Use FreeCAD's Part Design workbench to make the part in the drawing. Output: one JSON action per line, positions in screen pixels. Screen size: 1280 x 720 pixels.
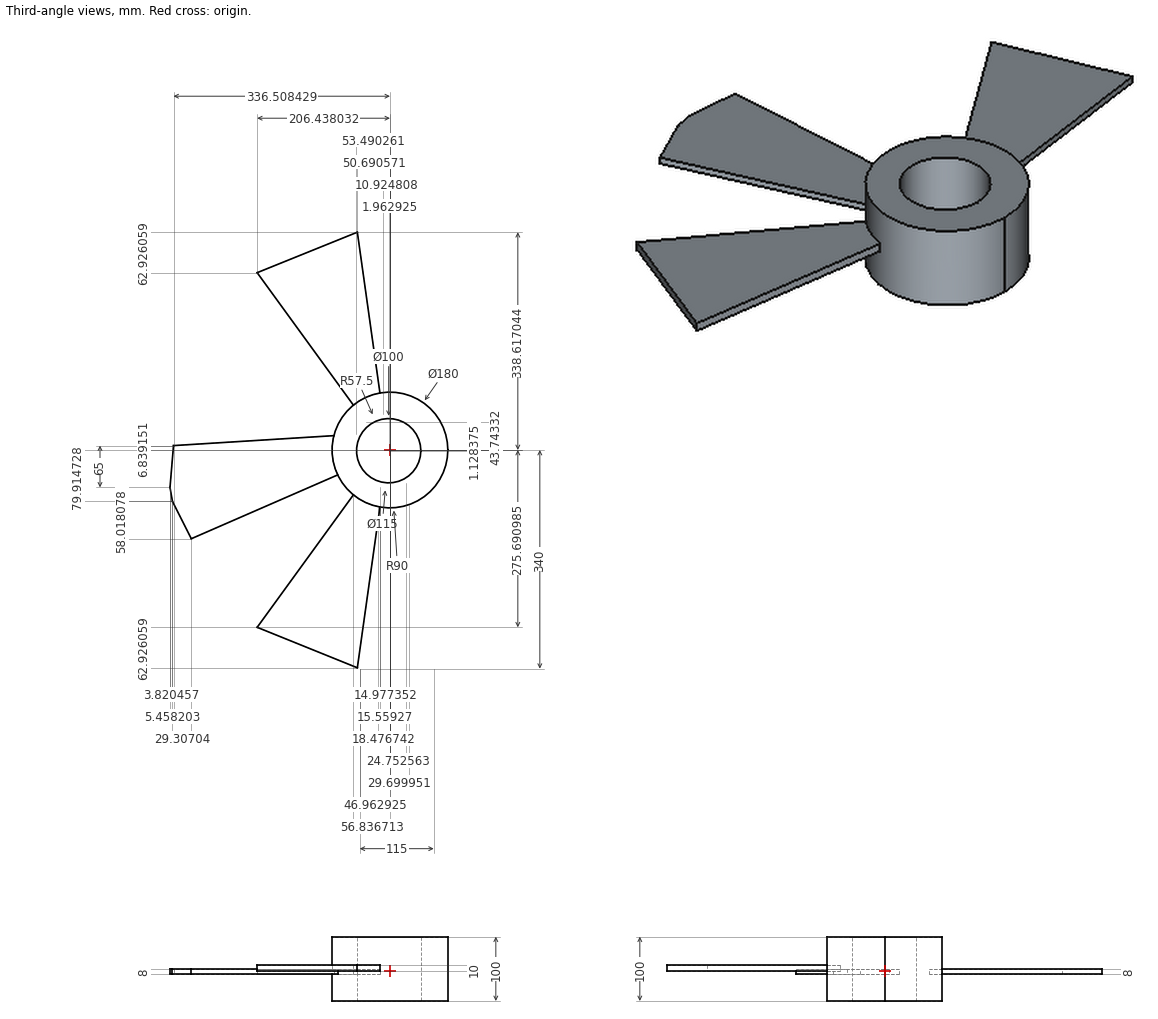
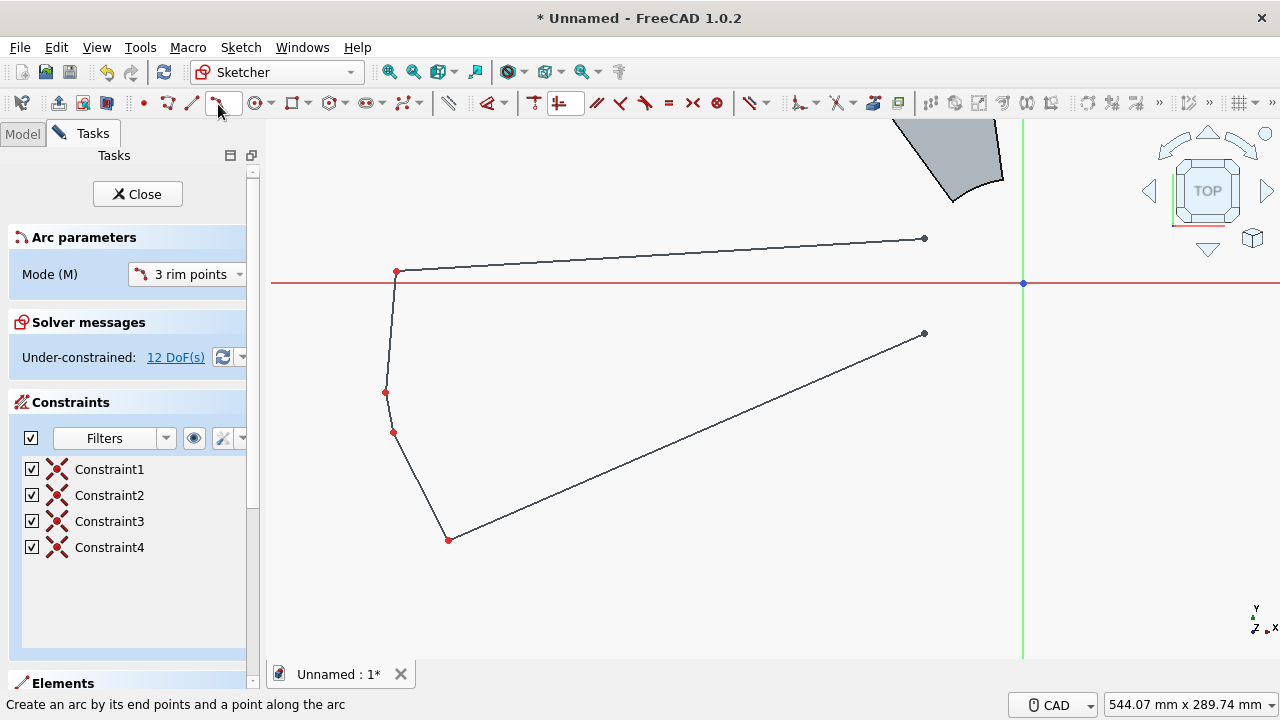
{"action": "left_click", "coordinate": [924, 334]}
{"action": "left_click", "coordinate": [924, 239]}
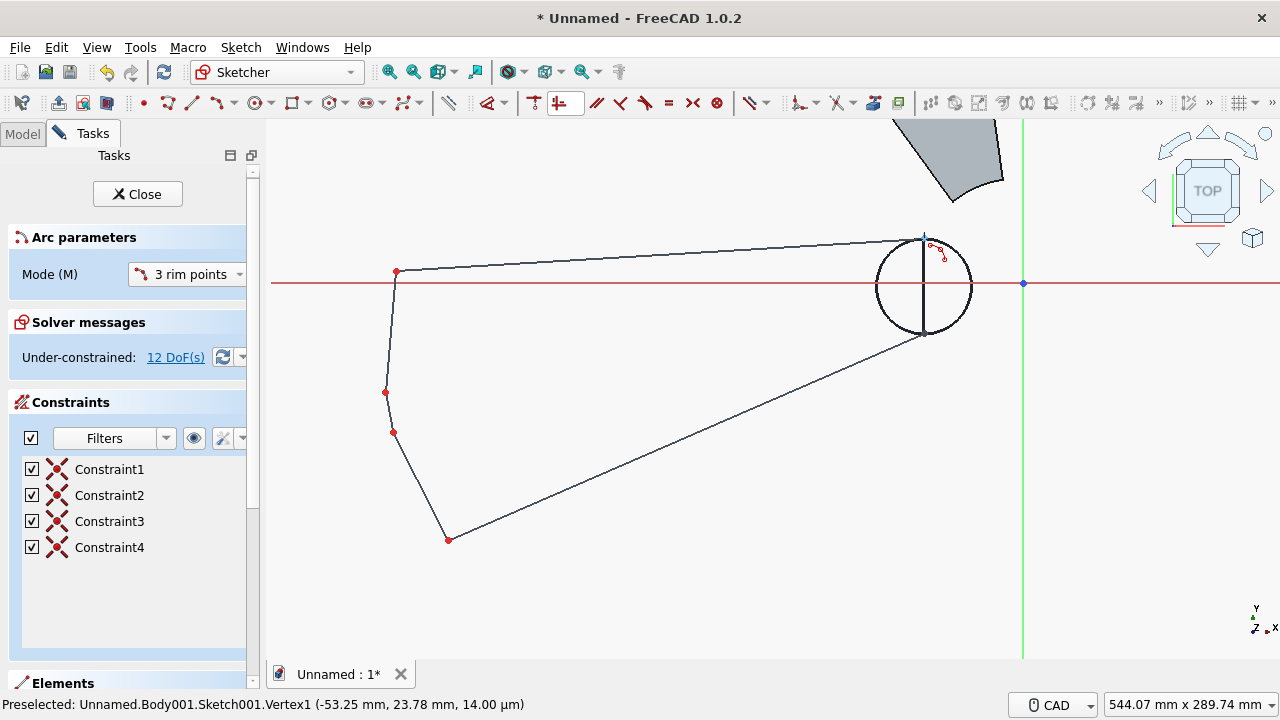
{"action": "scroll", "coordinate": [913, 295], "scroll_direction": "up", "scroll_amount": 2}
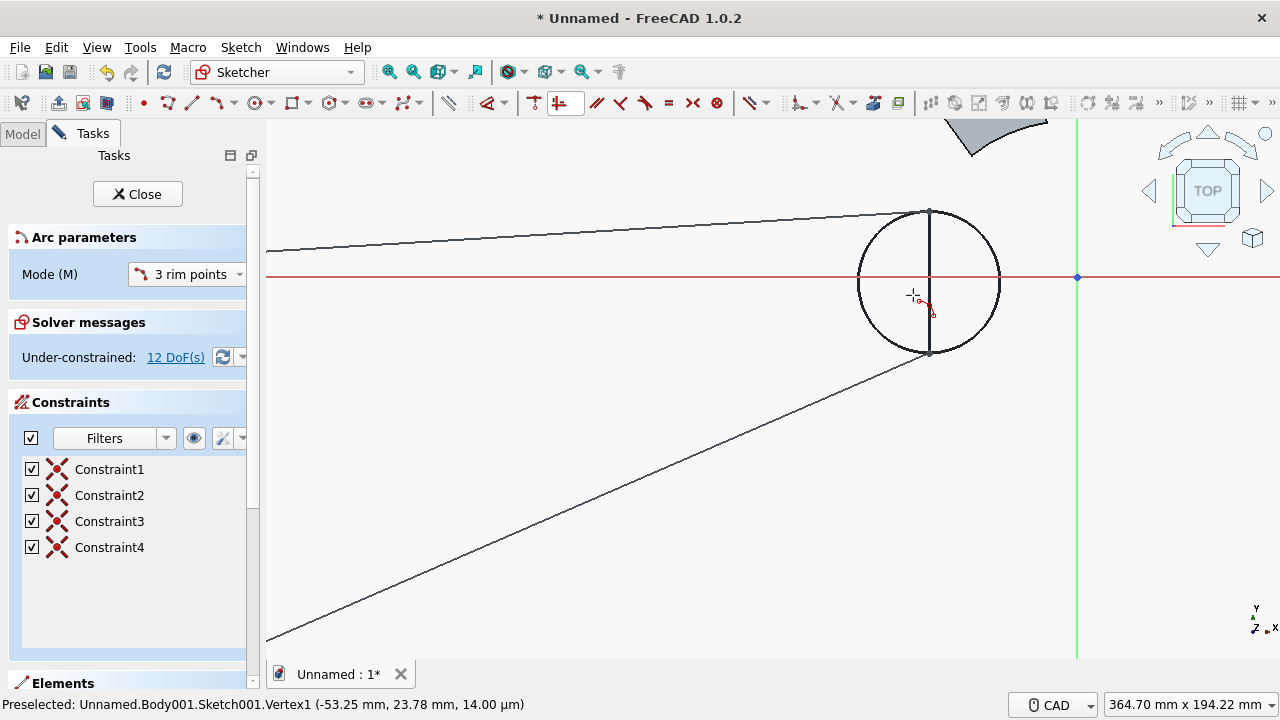
{"action": "left_click", "coordinate": [913, 295]}
{"action": "key", "text": "Escape"}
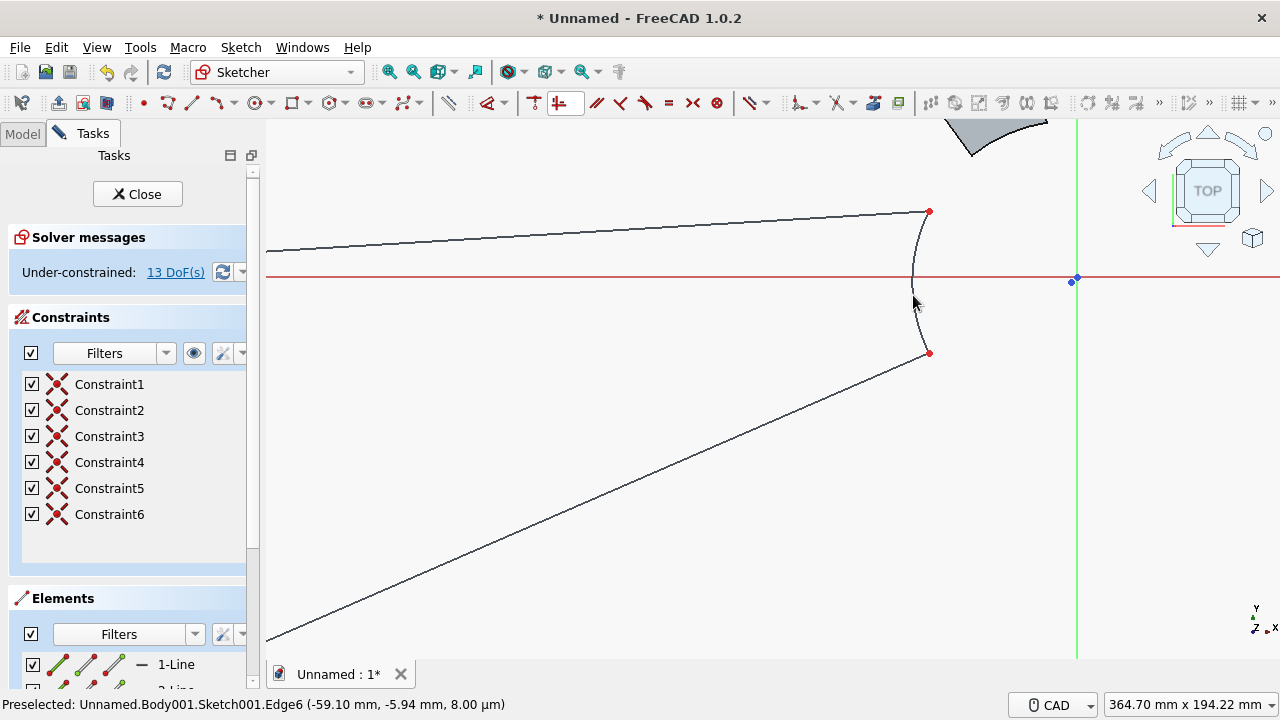
{"action": "left_click", "coordinate": [488, 104]}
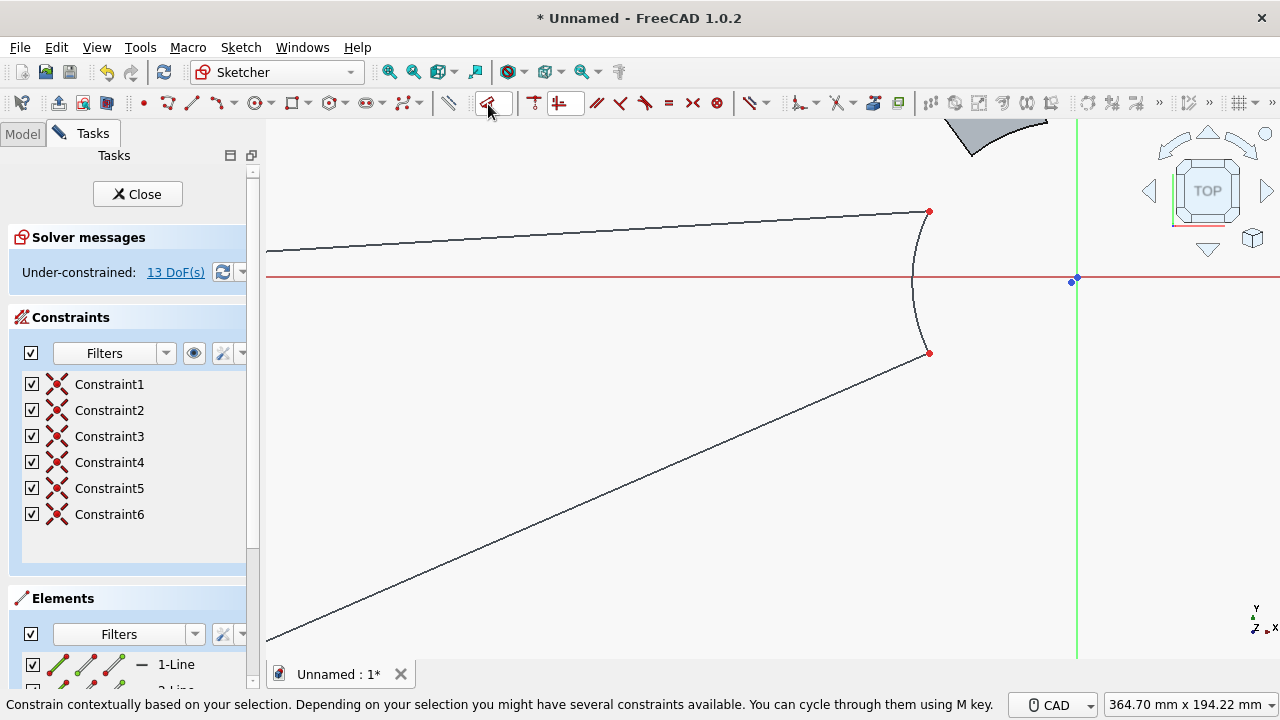
{"action": "left_click", "coordinate": [915, 253]}
{"action": "left_click", "coordinate": [884, 247]}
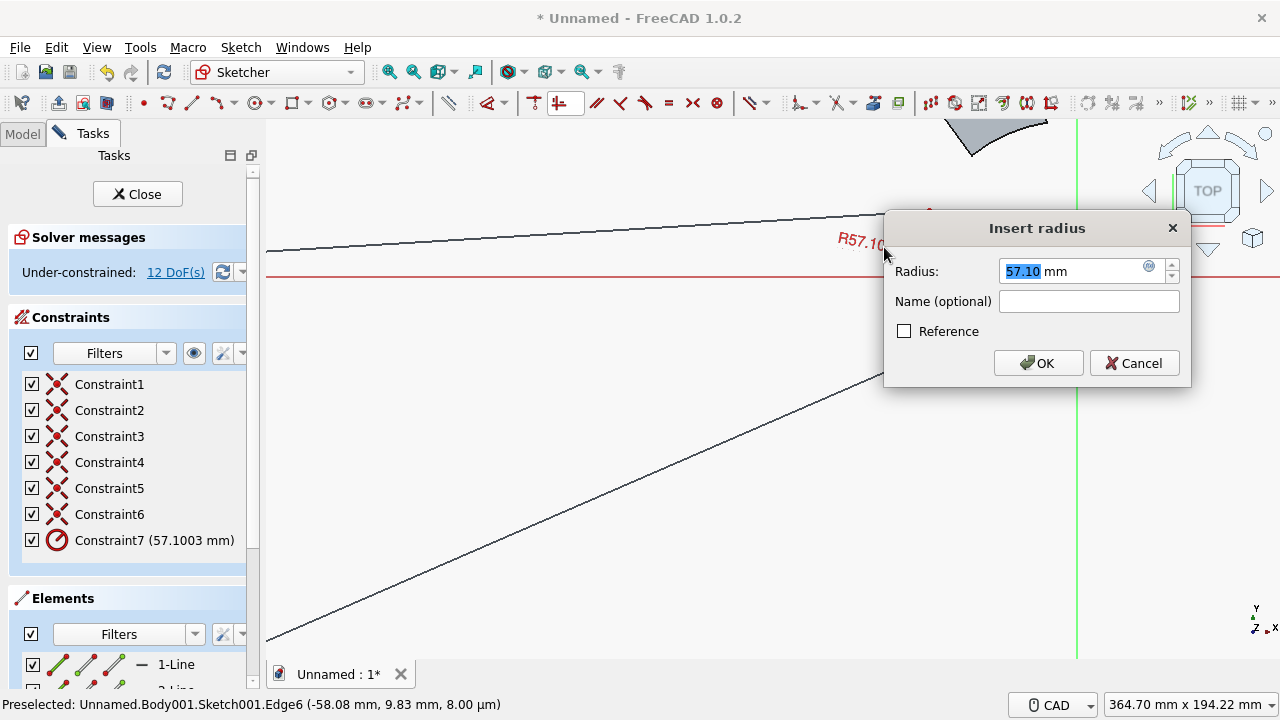
{"action": "type", "text": "57.5"}
{"action": "key", "text": "Return"}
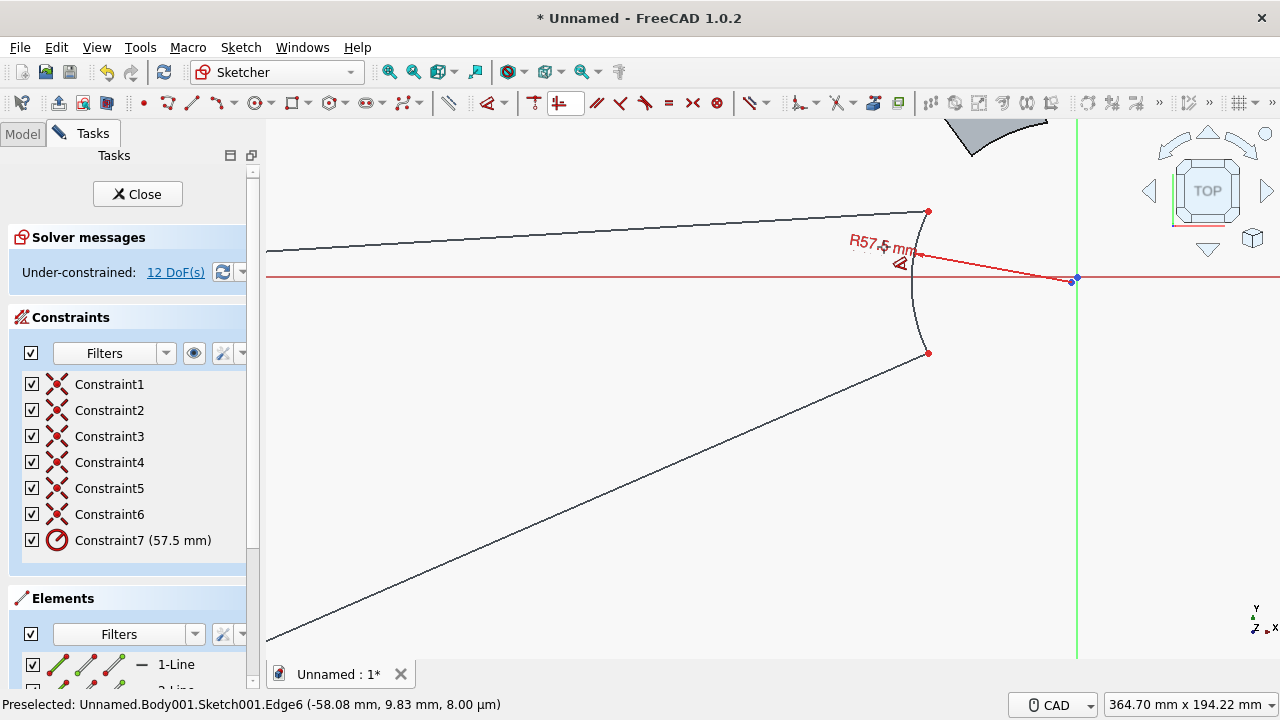
{"action": "scroll", "coordinate": [913, 295], "scroll_direction": "down", "scroll_amount": 2}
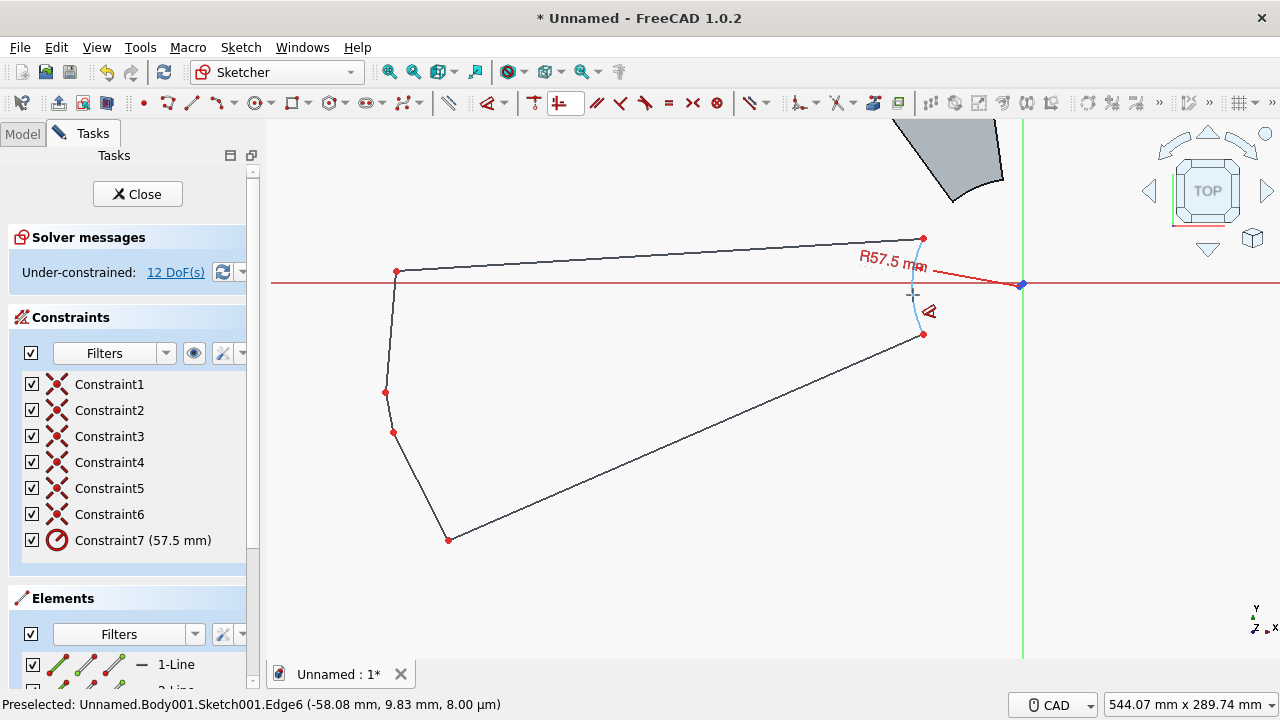
{"action": "left_click", "coordinate": [393, 307]}
{"action": "left_click", "coordinate": [352, 332]}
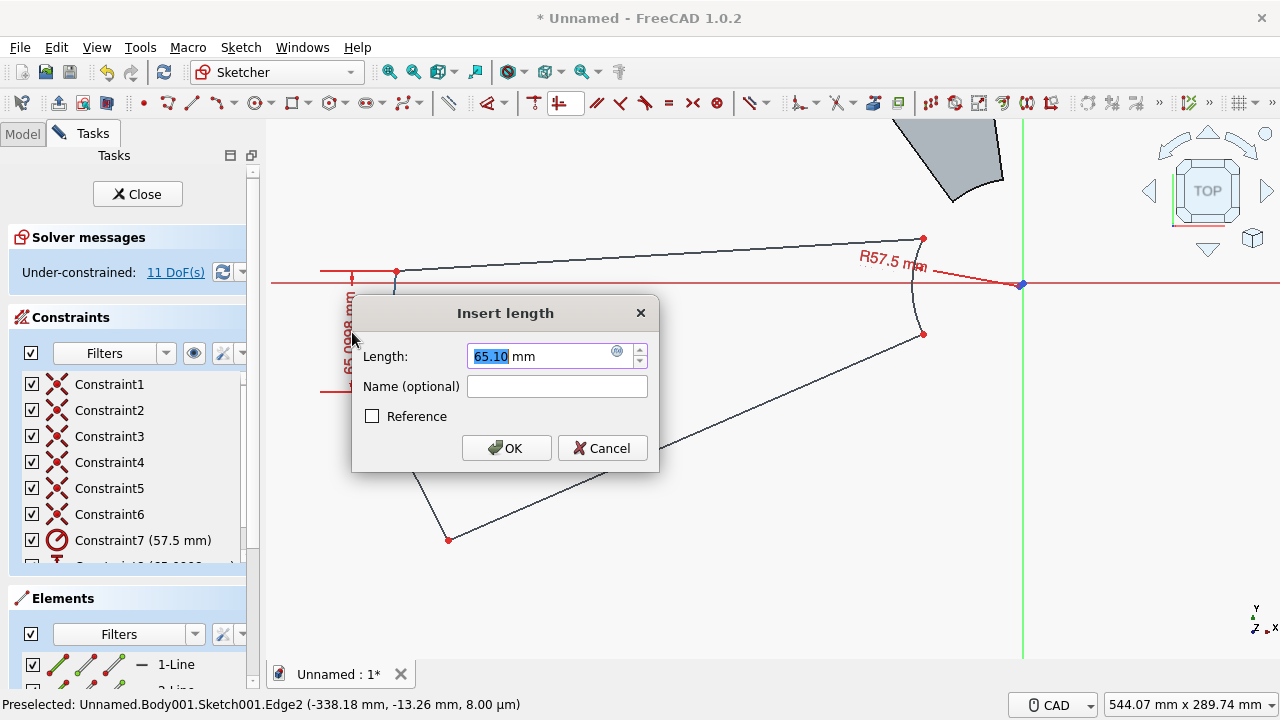
{"action": "type", "text": "65"}
{"action": "key", "text": "Return"}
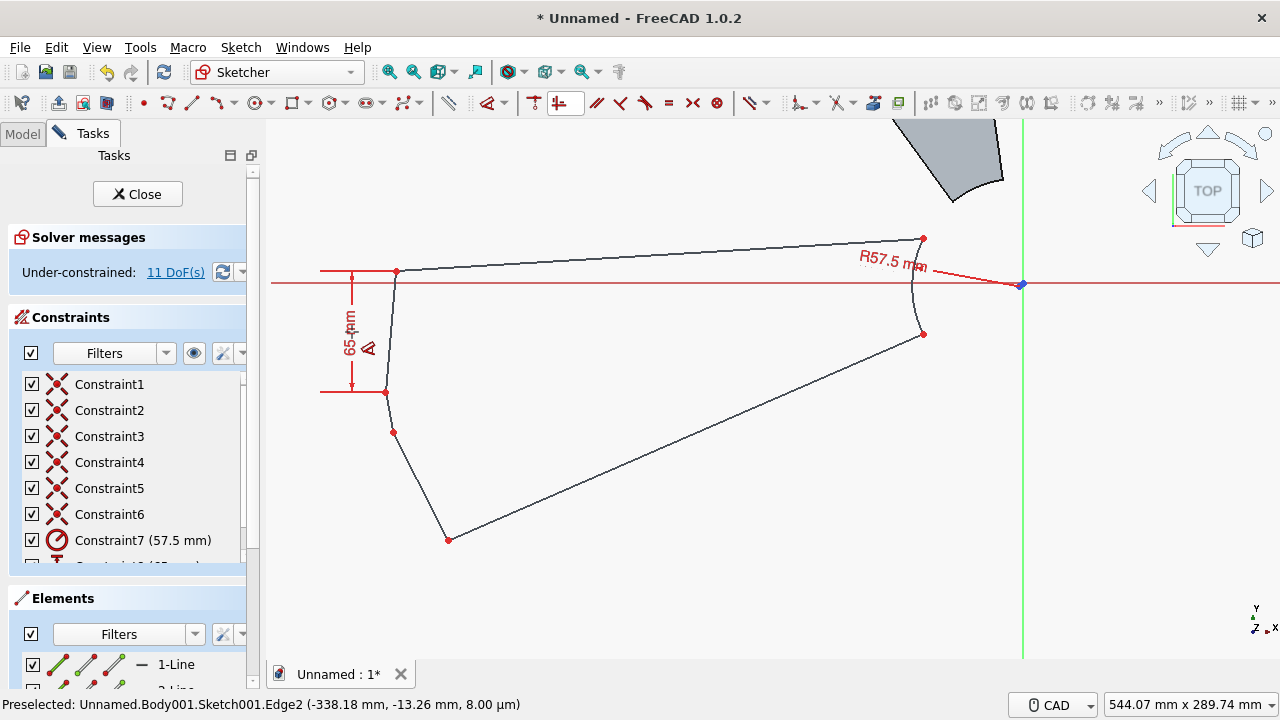
{"action": "scroll", "coordinate": [396, 271], "scroll_direction": "up", "scroll_amount": 6}